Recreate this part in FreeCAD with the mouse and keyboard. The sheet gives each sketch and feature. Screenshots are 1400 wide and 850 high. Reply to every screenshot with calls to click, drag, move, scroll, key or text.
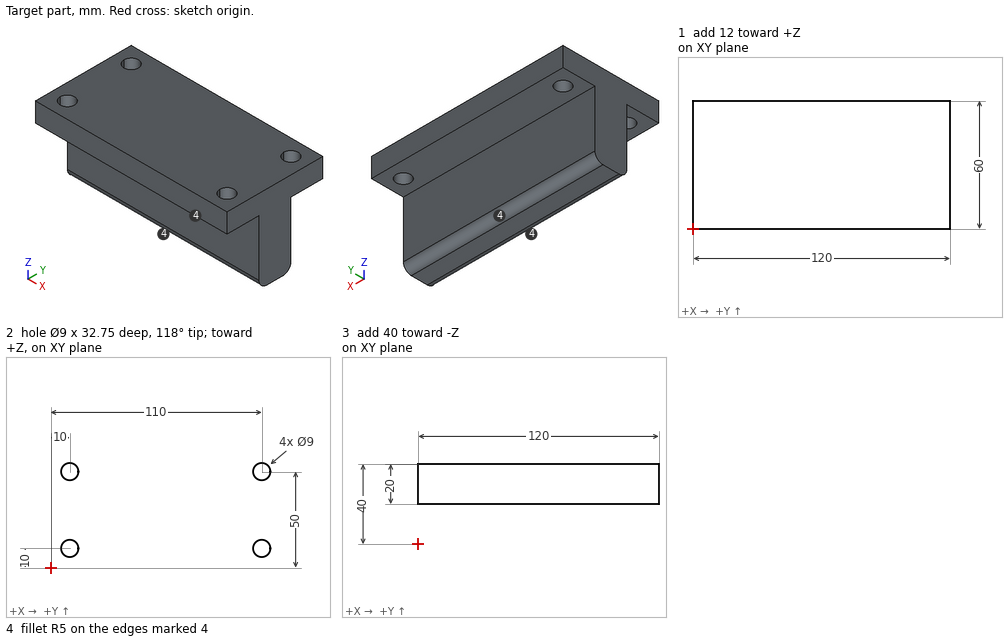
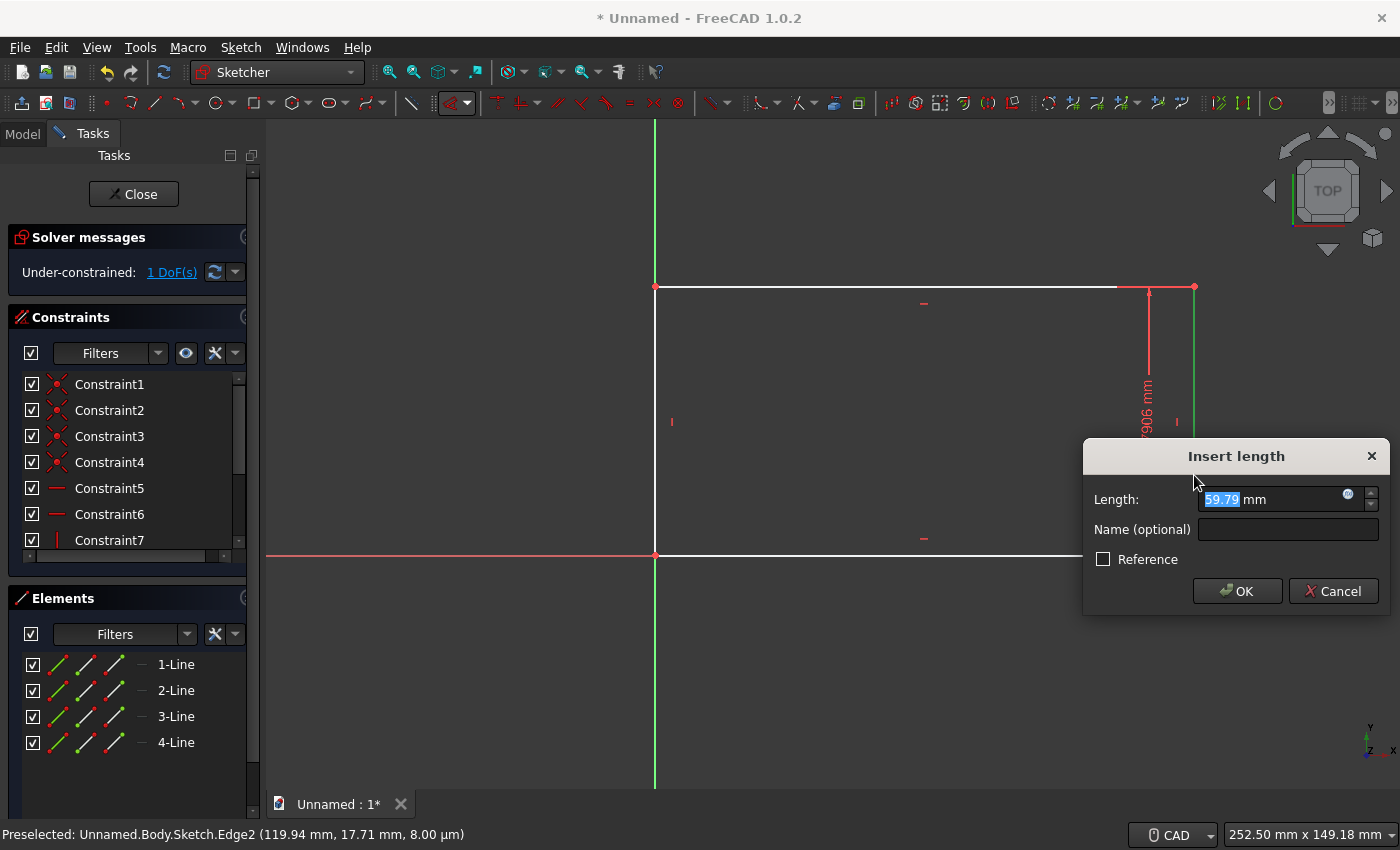
text(60)
key(Return)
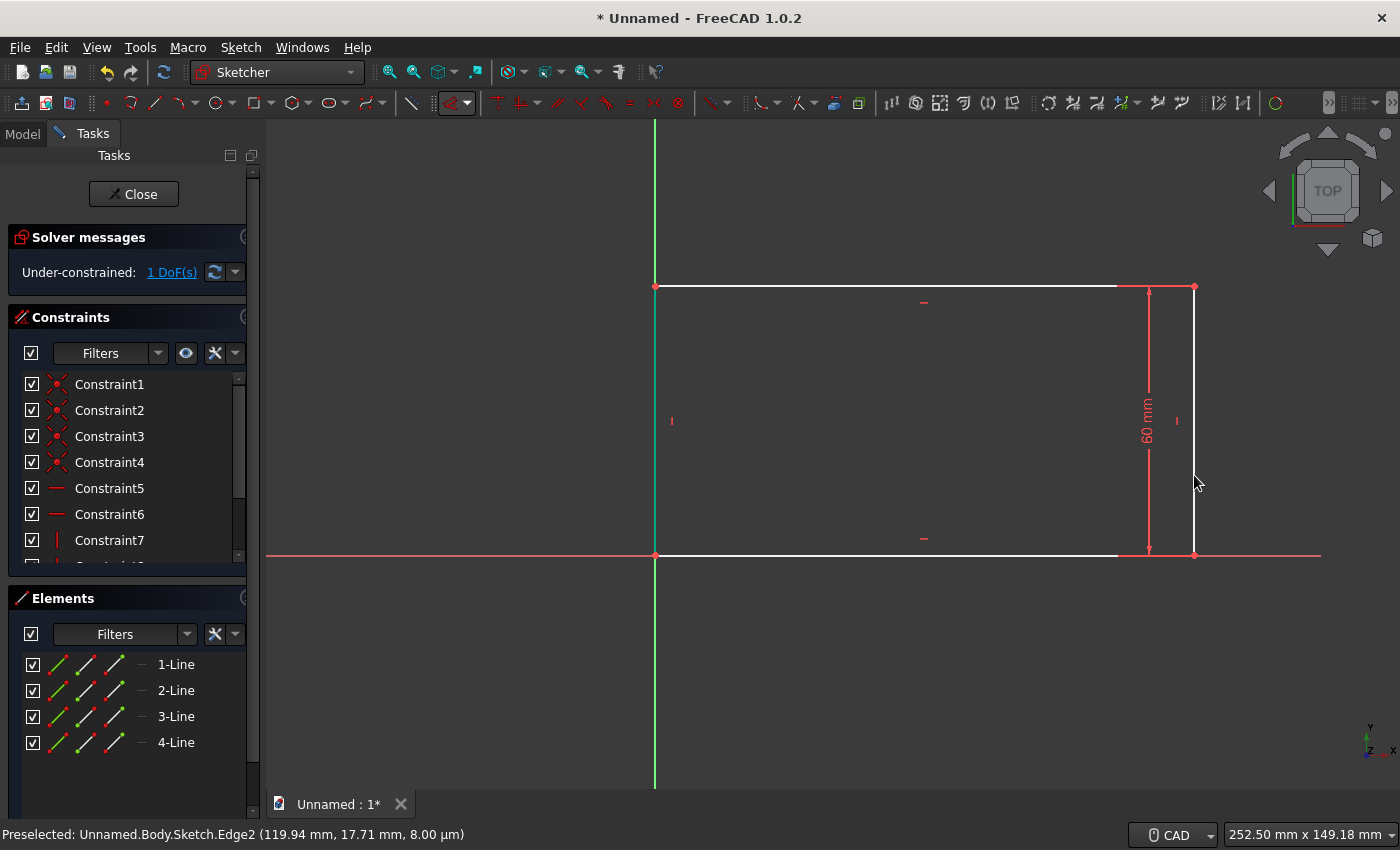
click(817, 556)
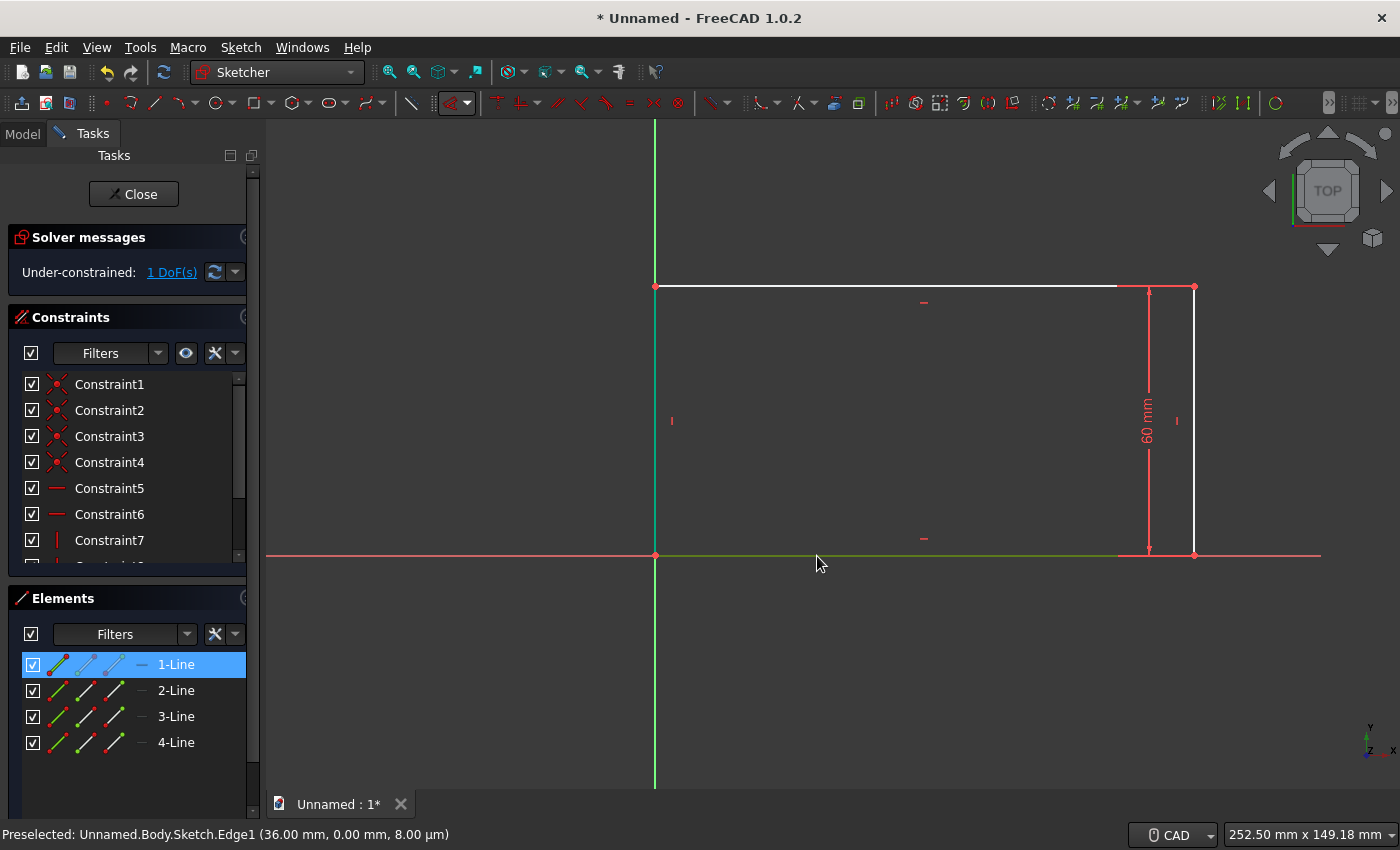
click(470, 104)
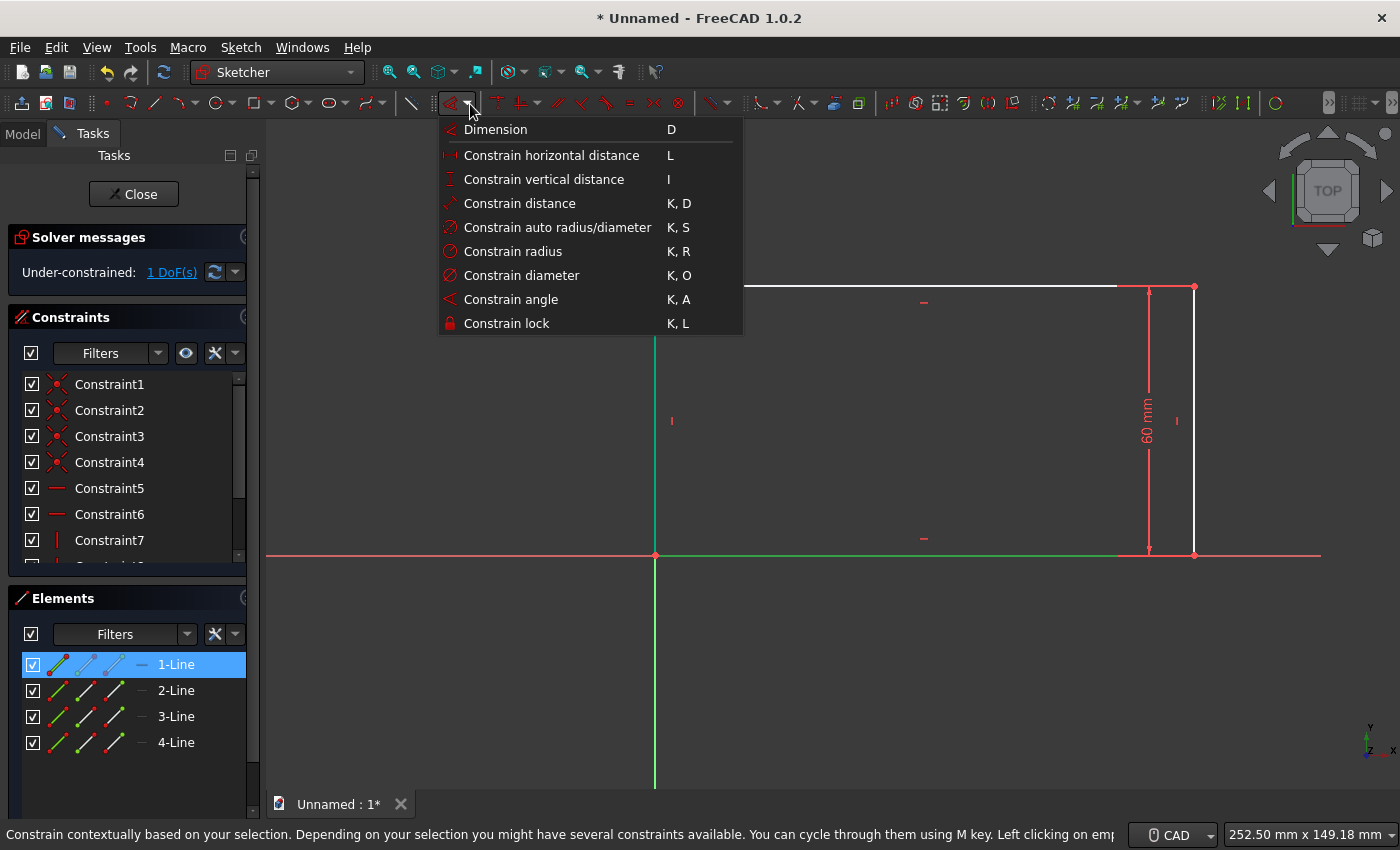
click(591, 155)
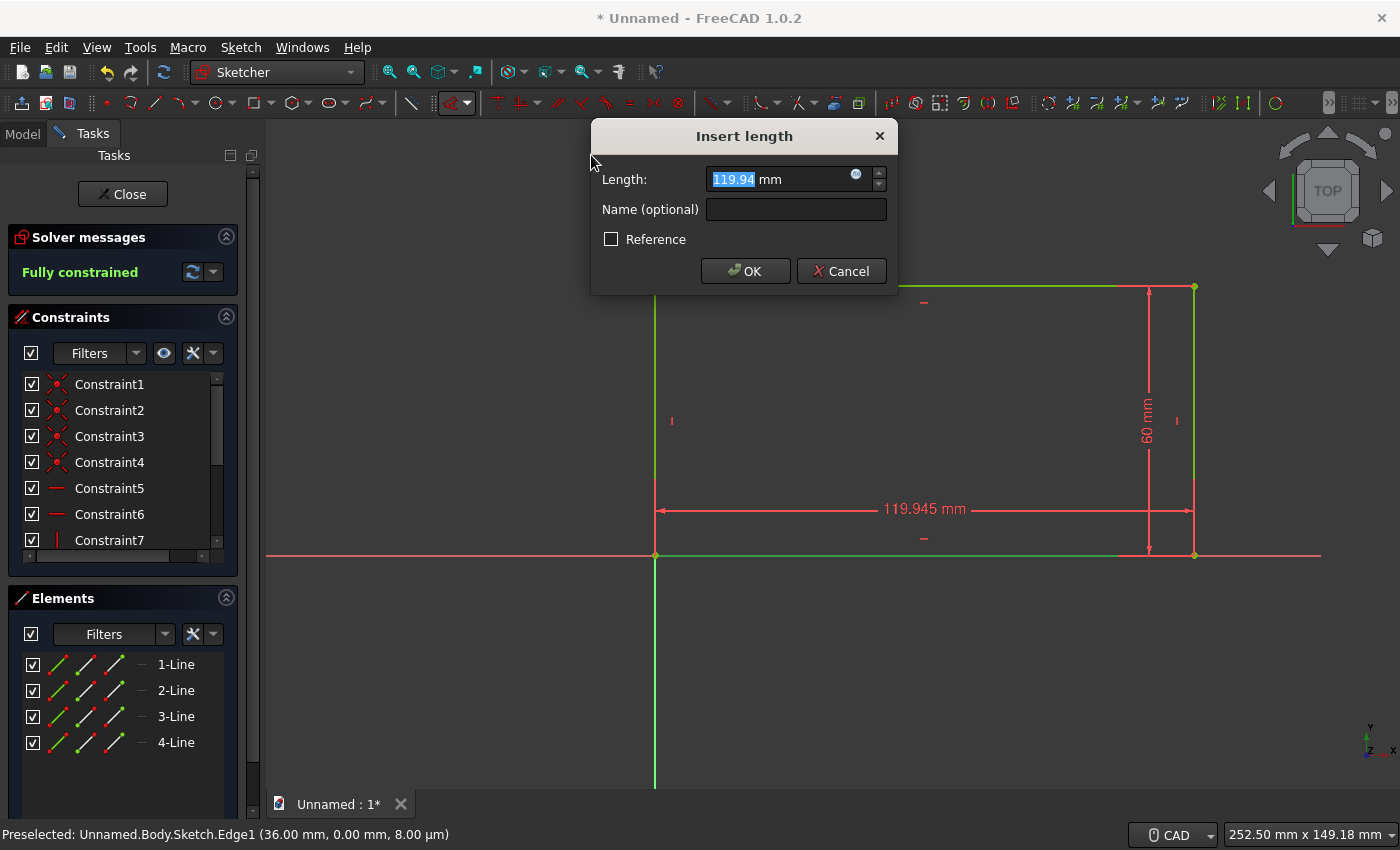
text(120)
key(Return)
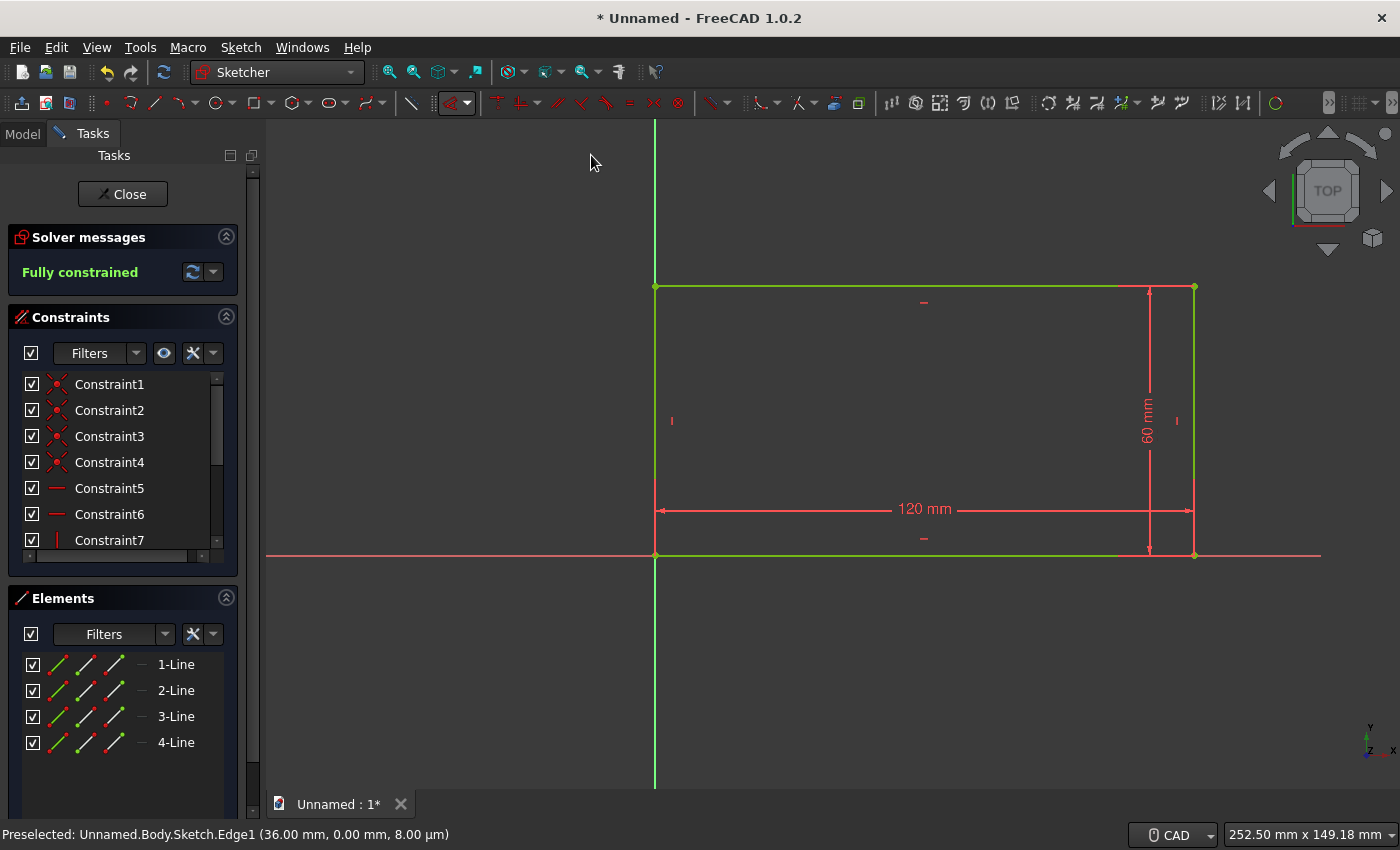
click(123, 194)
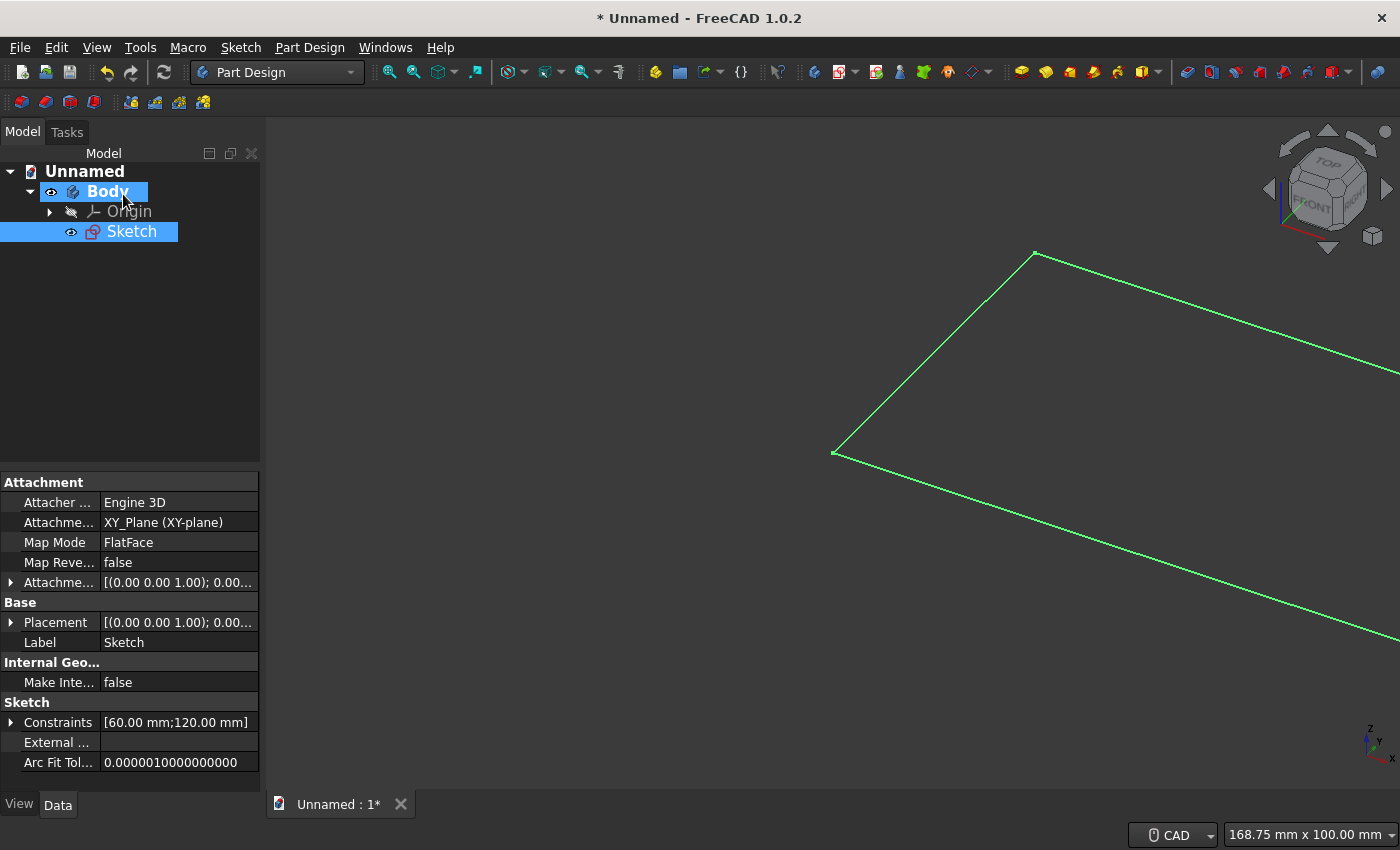
click(1022, 72)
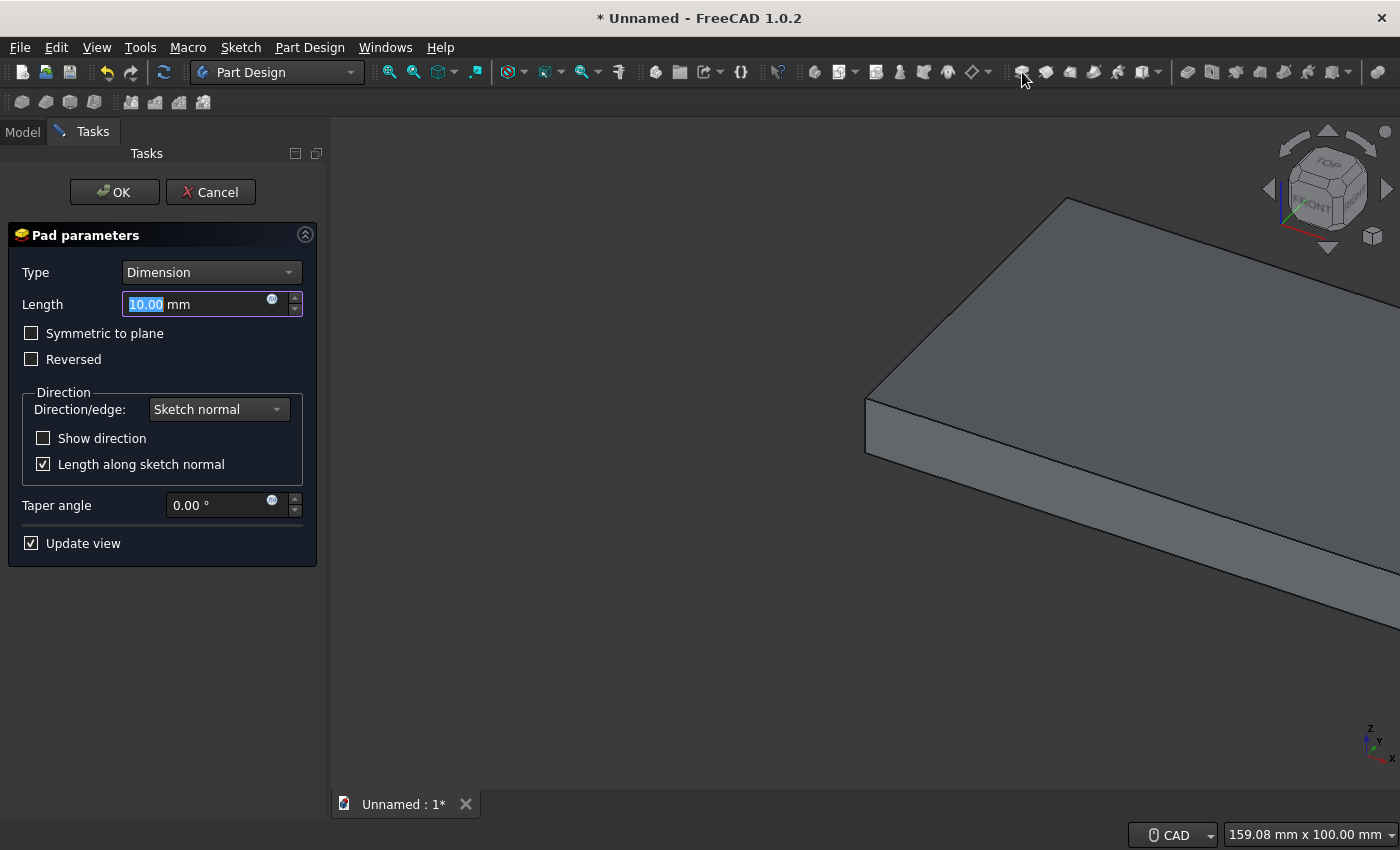
text(12)
key(Tab)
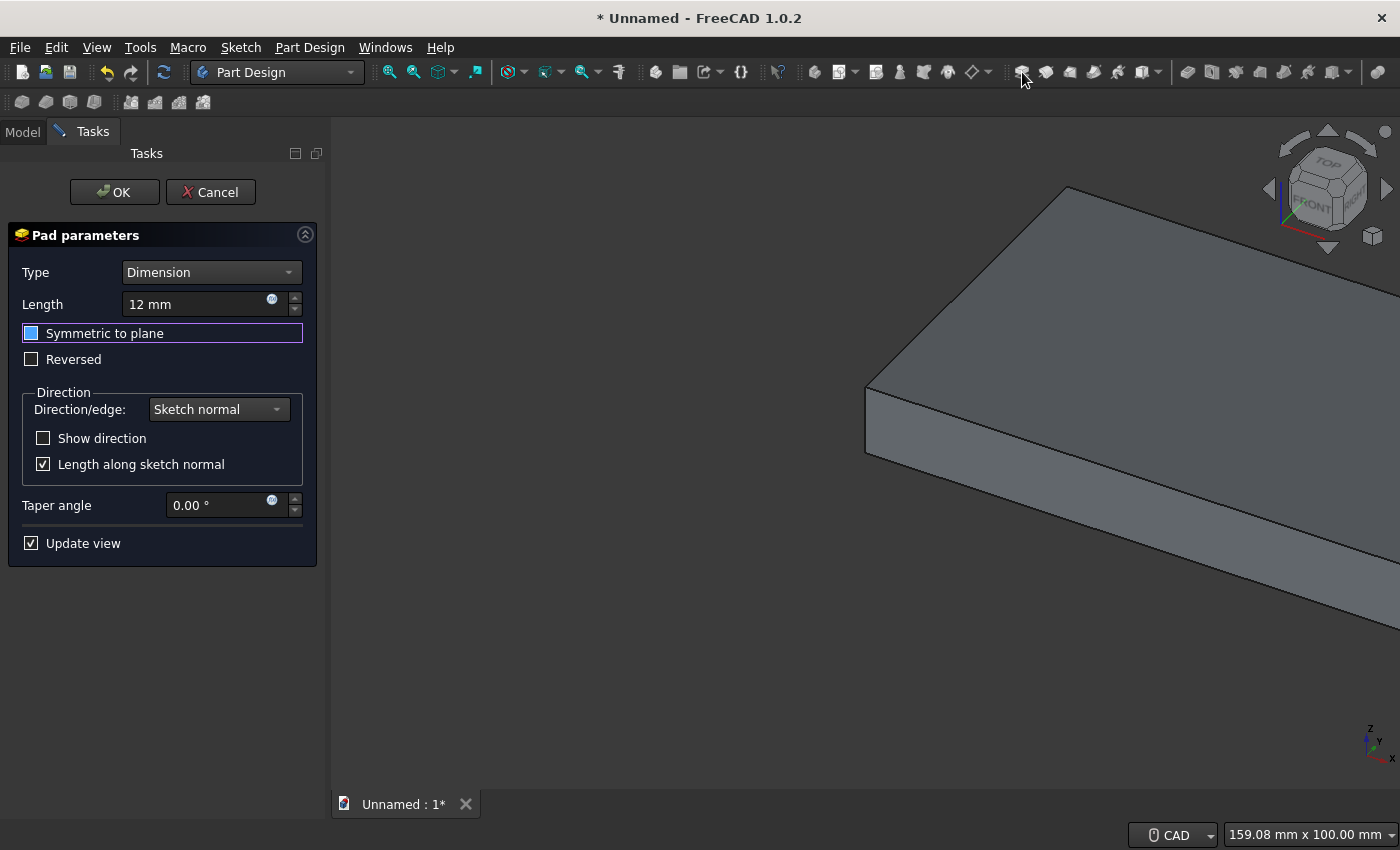
click(115, 192)